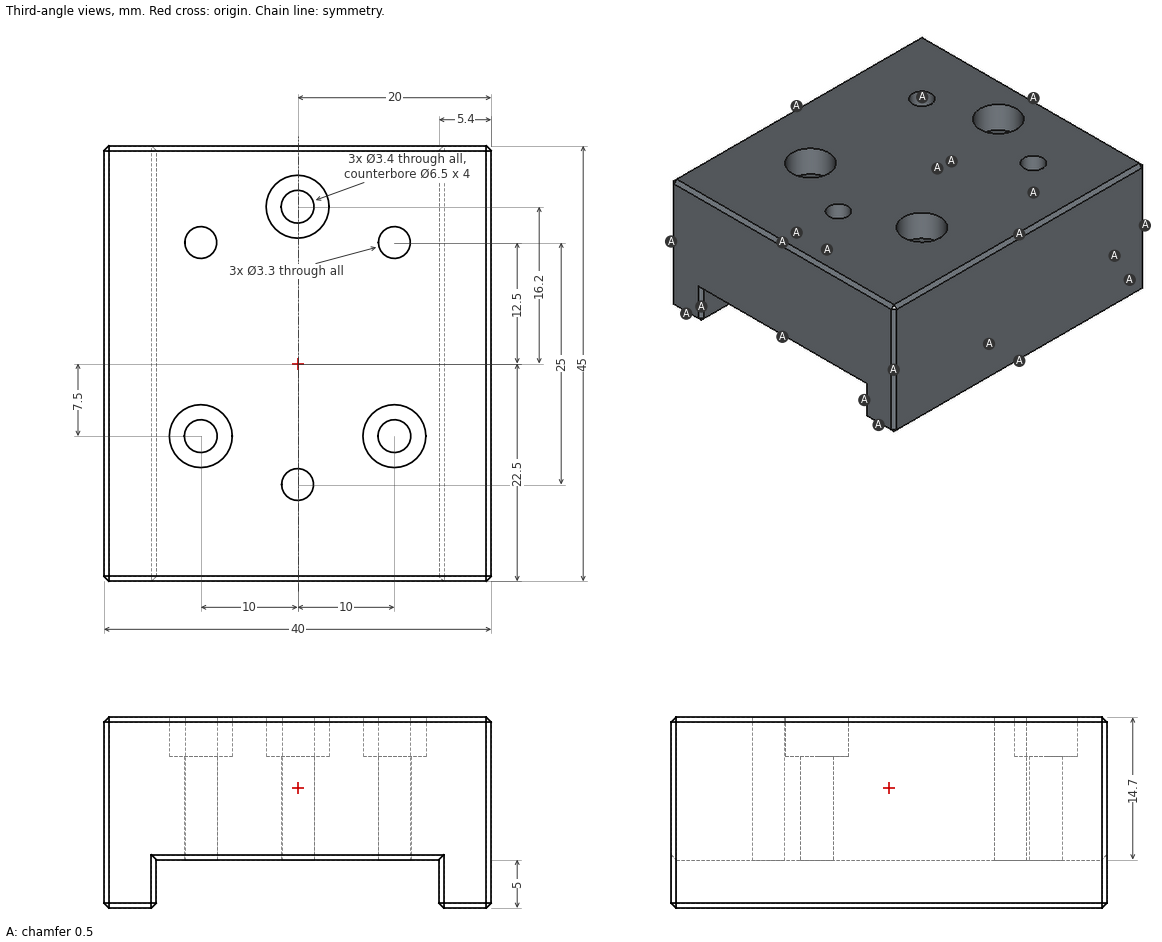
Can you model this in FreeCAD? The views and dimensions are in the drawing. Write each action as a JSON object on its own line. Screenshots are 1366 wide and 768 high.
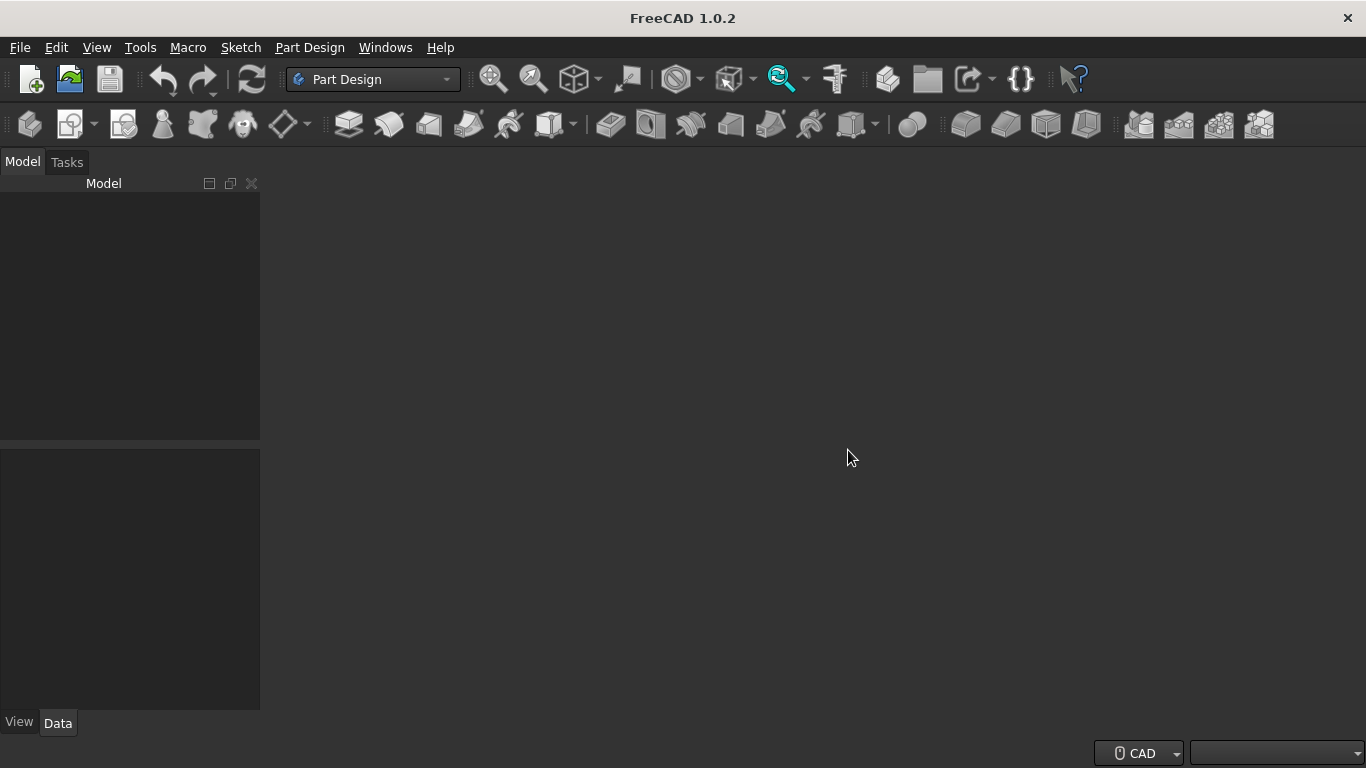
{"action": "left_click", "coordinate": [30, 80]}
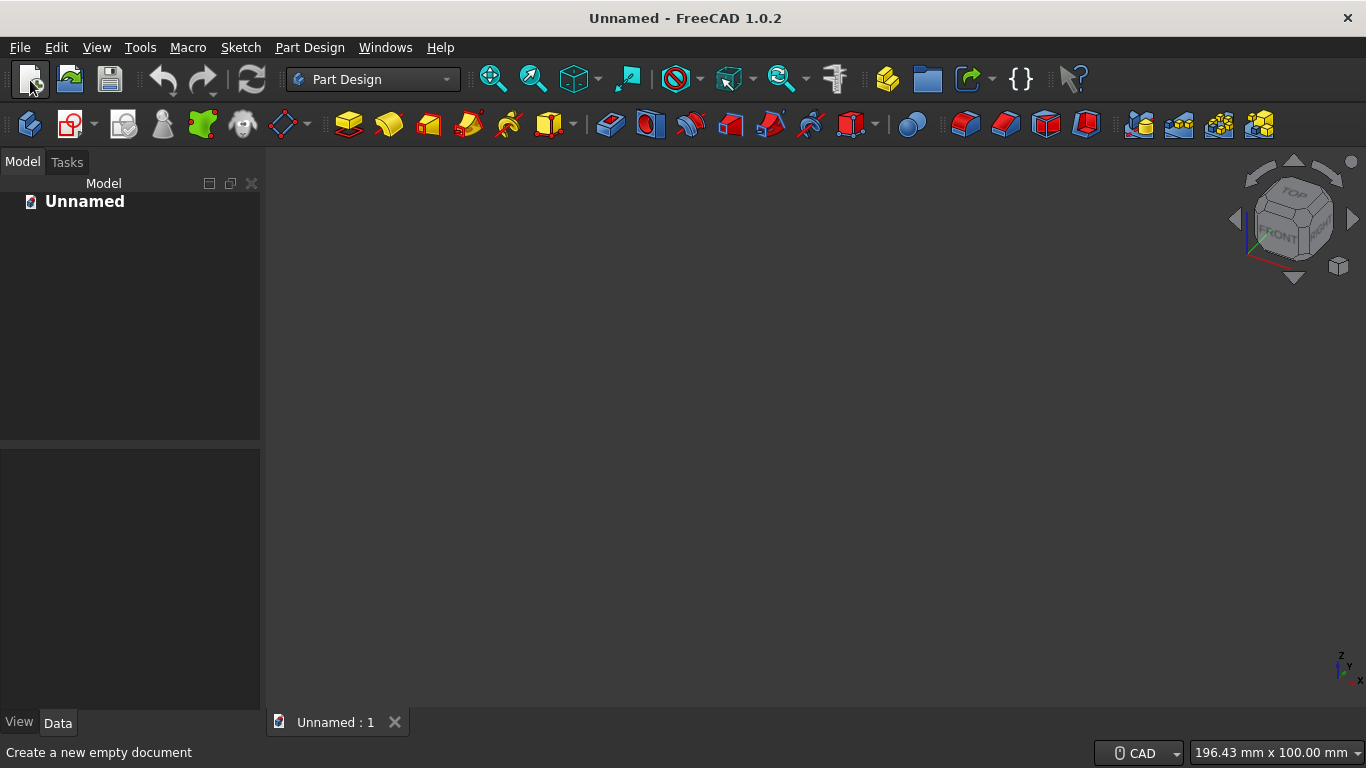
{"action": "left_click", "coordinate": [70, 124]}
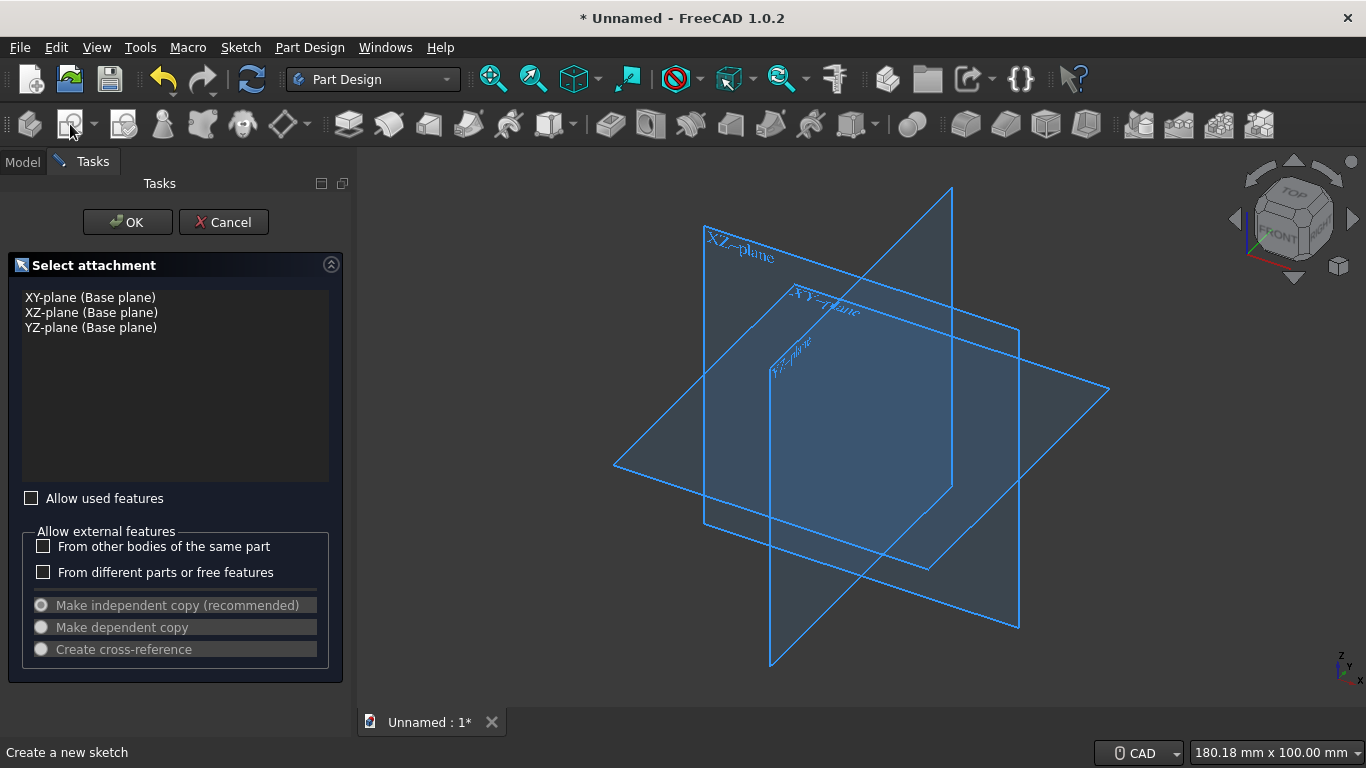
{"action": "left_click", "coordinate": [82, 298]}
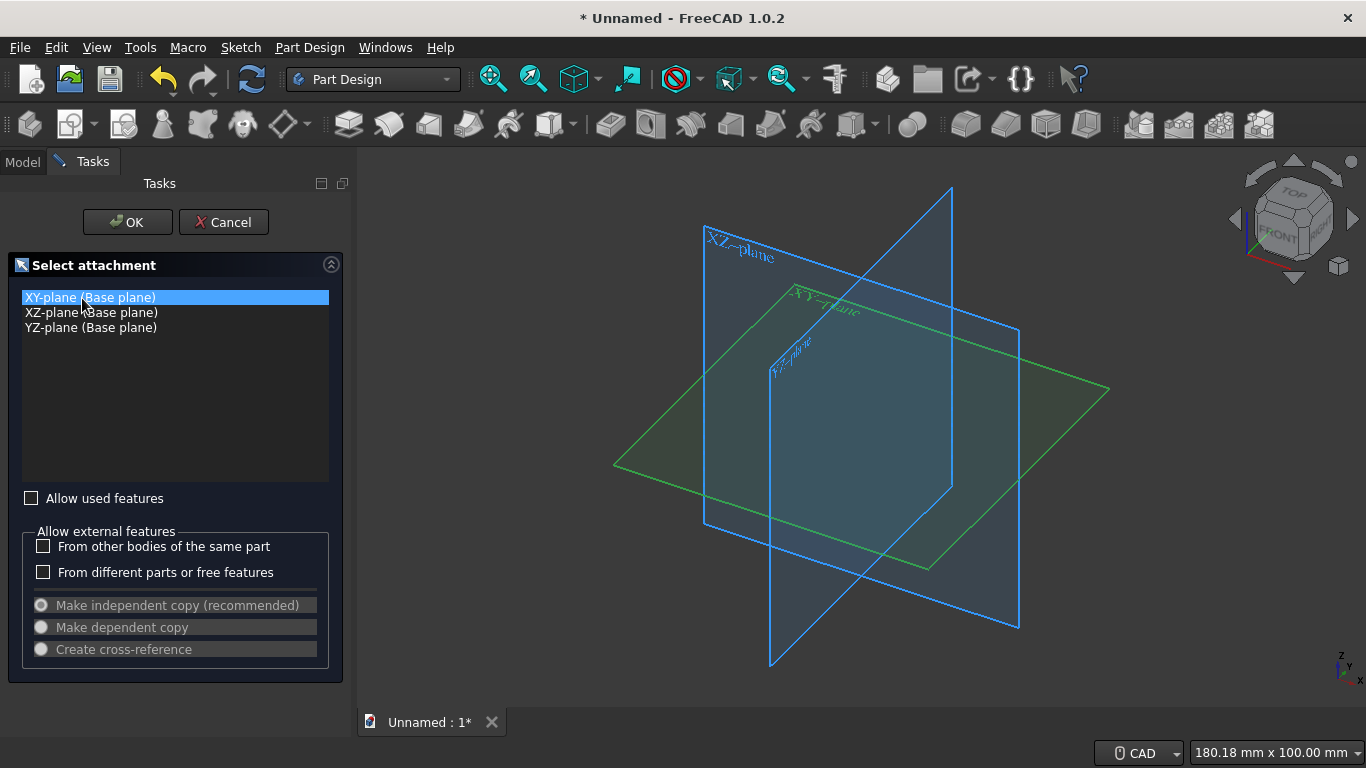
{"action": "left_click", "coordinate": [128, 222]}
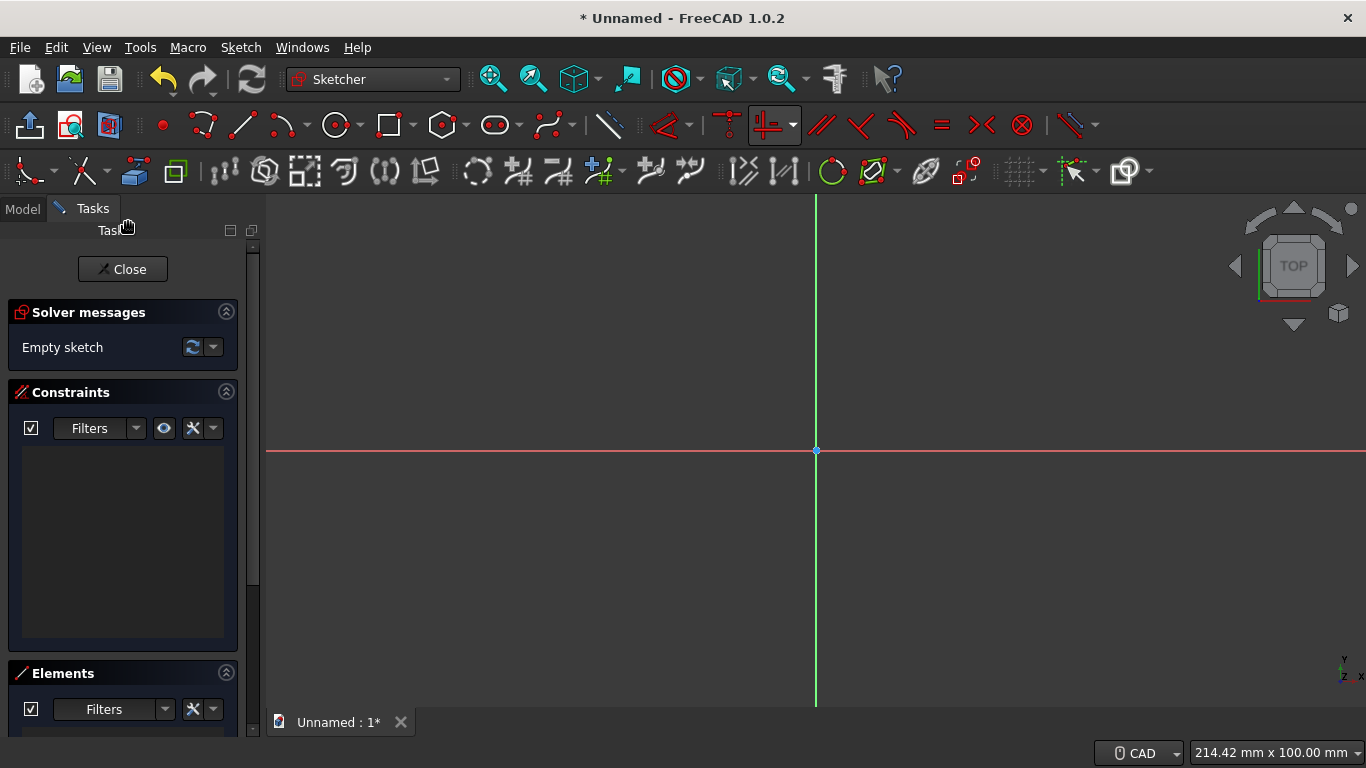
{"action": "scroll", "coordinate": [955, 451], "scroll_direction": "up", "scroll_amount": 2}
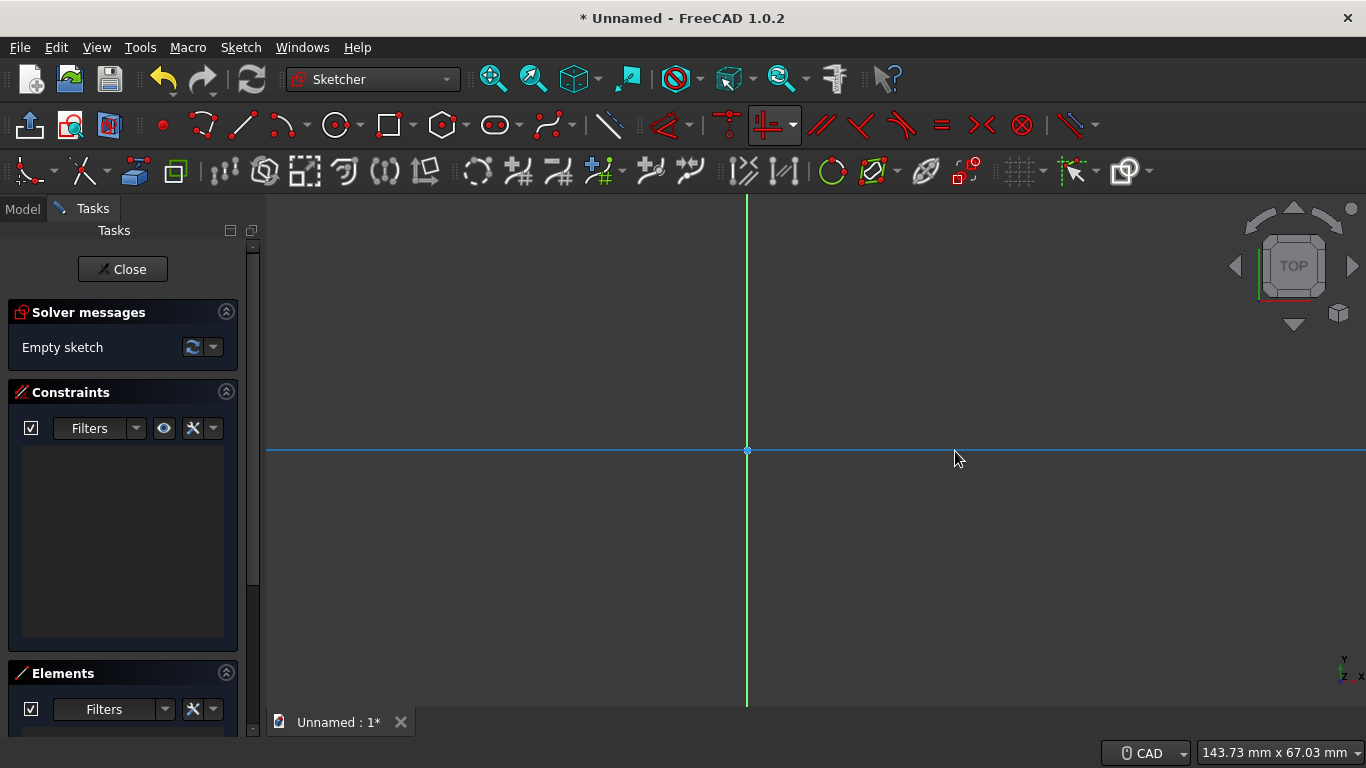
{"action": "key", "text": "g v"}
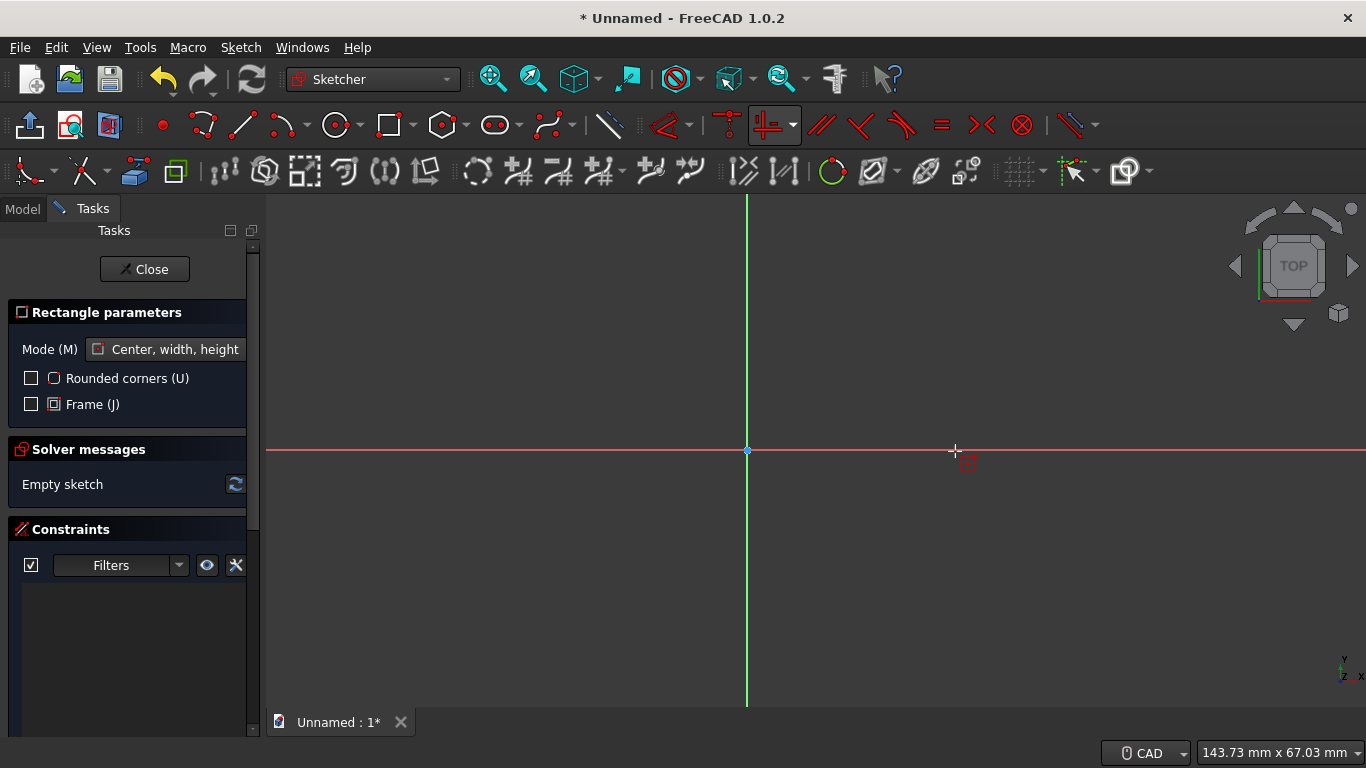
{"action": "left_click", "coordinate": [747, 450]}
{"action": "left_click", "coordinate": [900, 278]}
{"action": "key", "text": "Escape"}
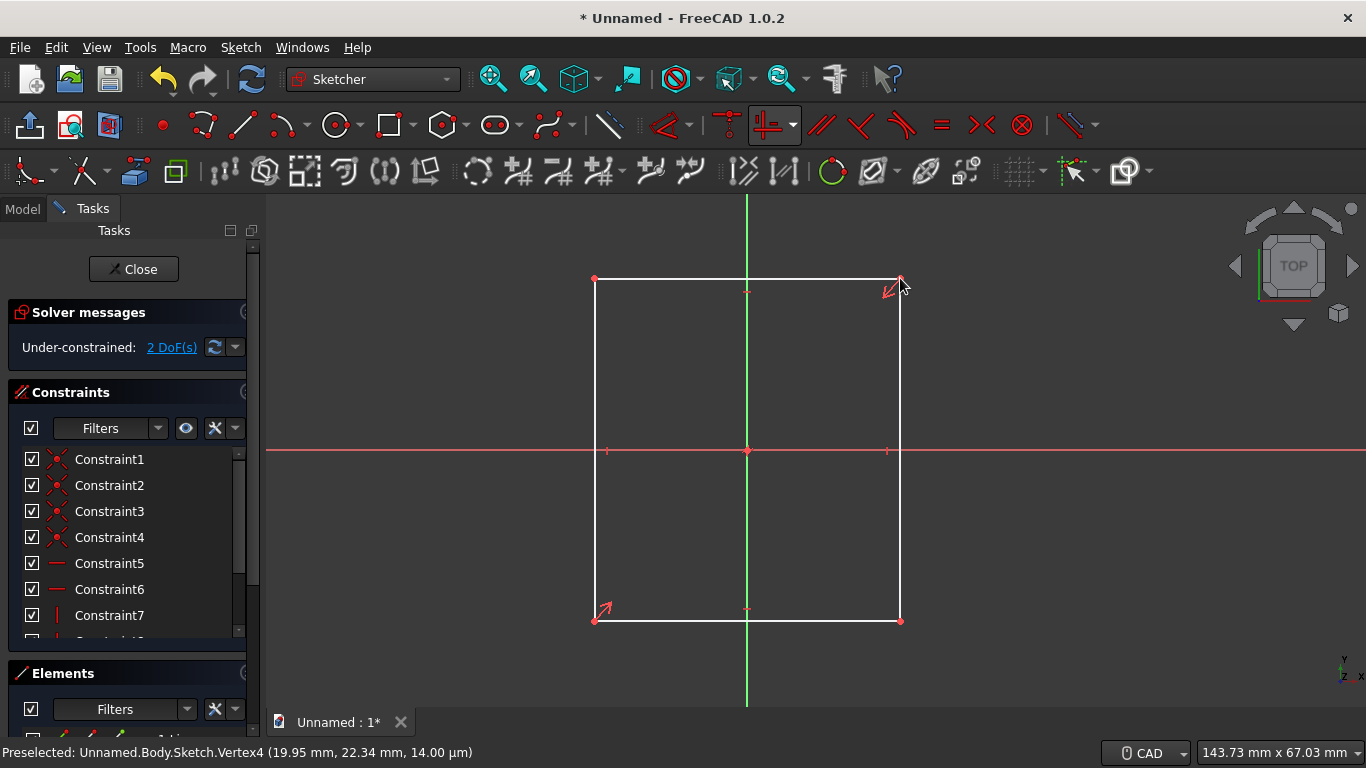
{"action": "left_click", "coordinate": [686, 621]}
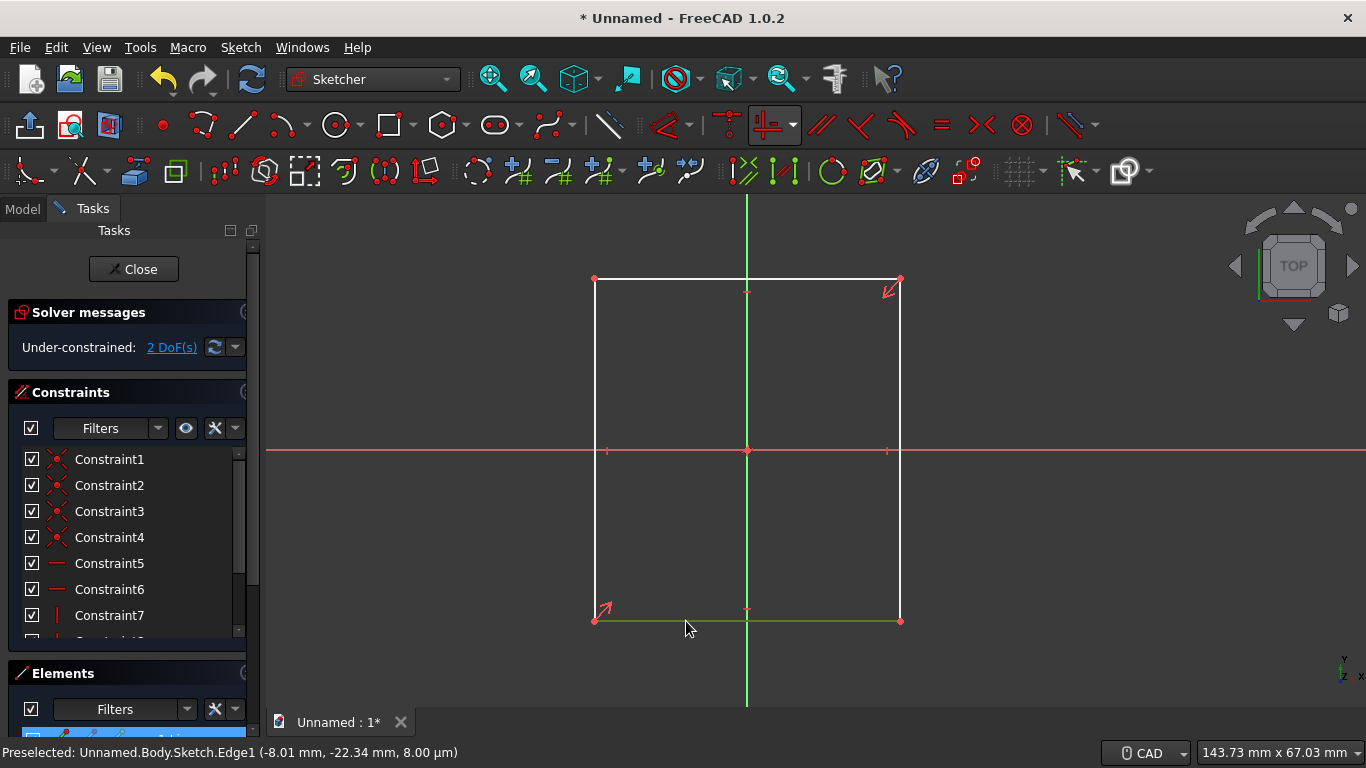
{"action": "key", "text": "l"}